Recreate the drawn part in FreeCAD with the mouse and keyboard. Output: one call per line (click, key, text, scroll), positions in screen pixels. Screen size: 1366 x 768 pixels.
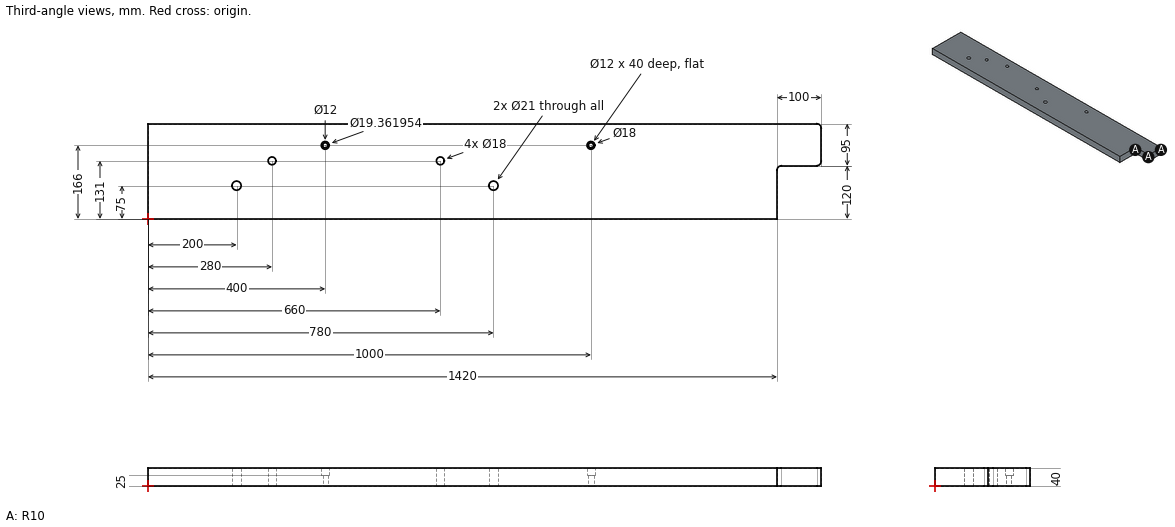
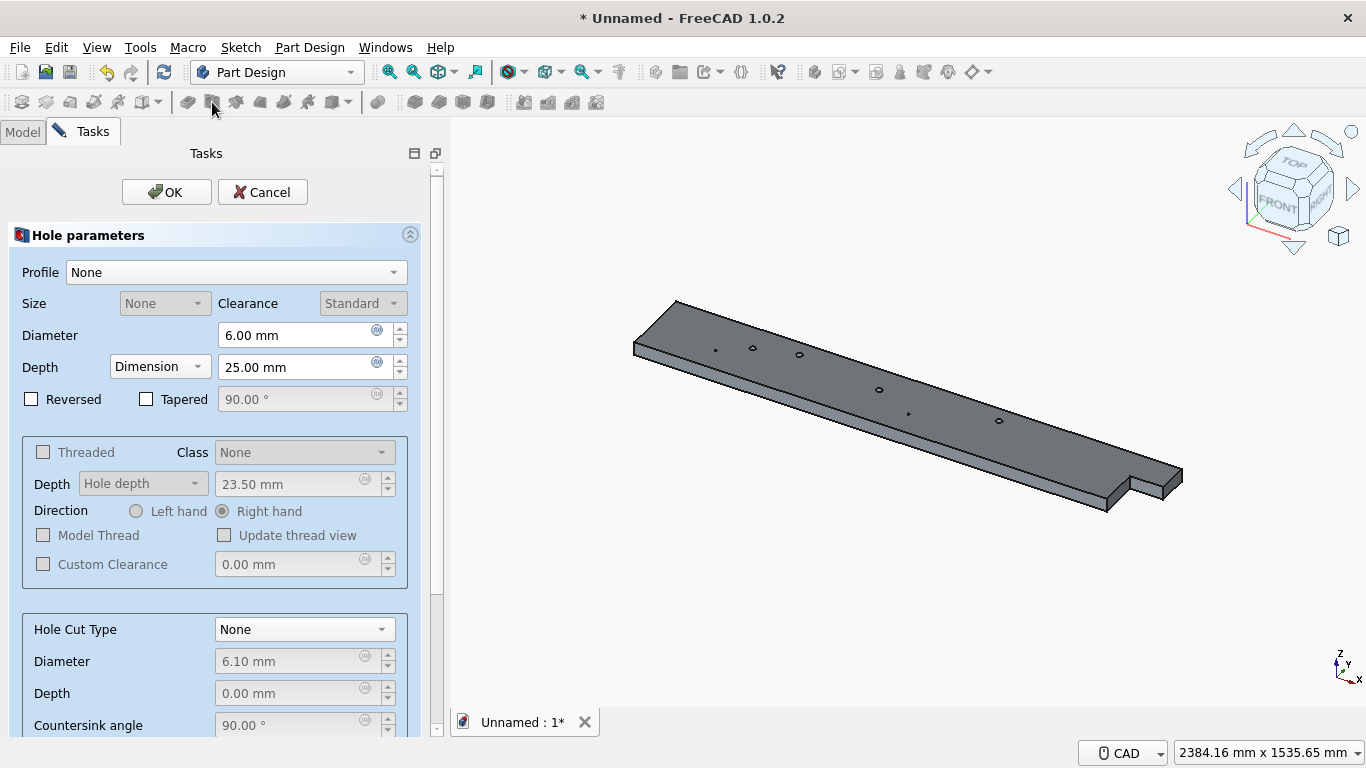
triple_click(305, 335)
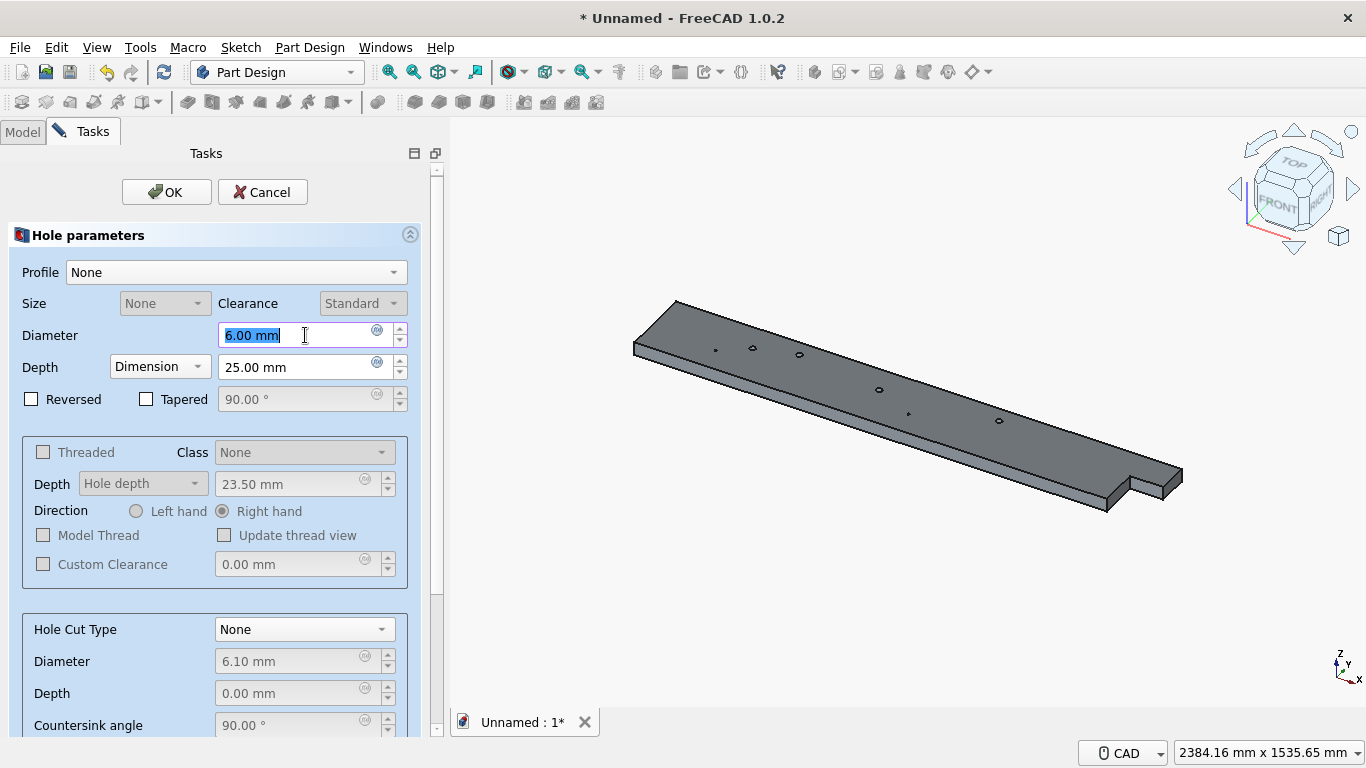
text(21)
key(Tab)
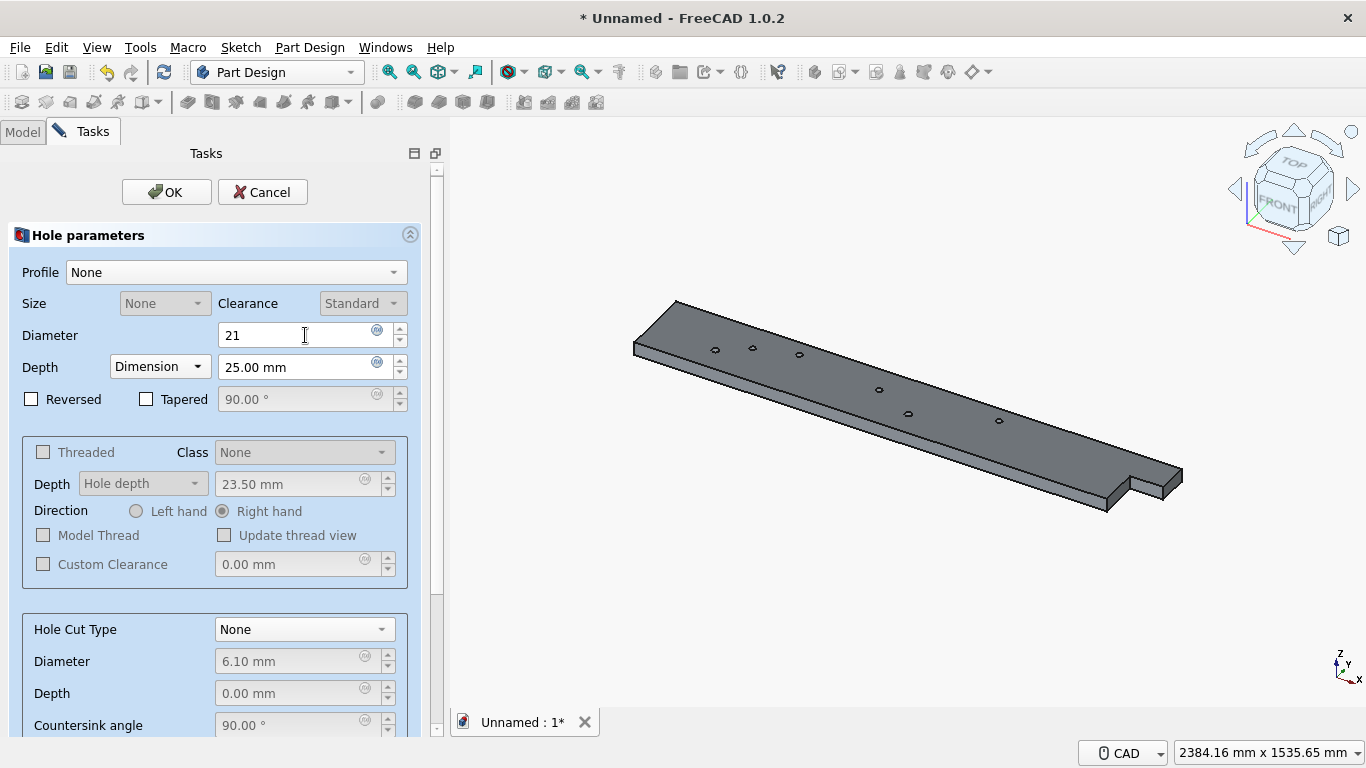
click(161, 366)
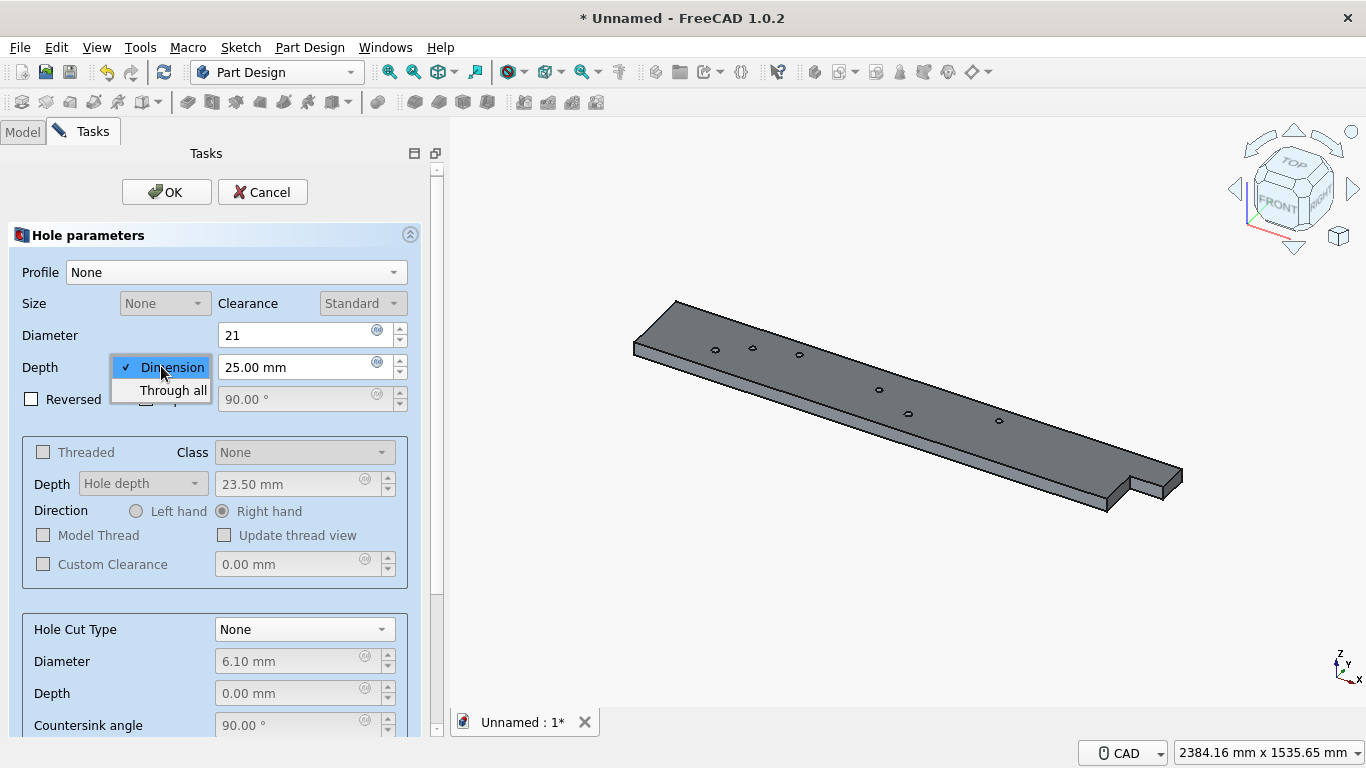
click(160, 390)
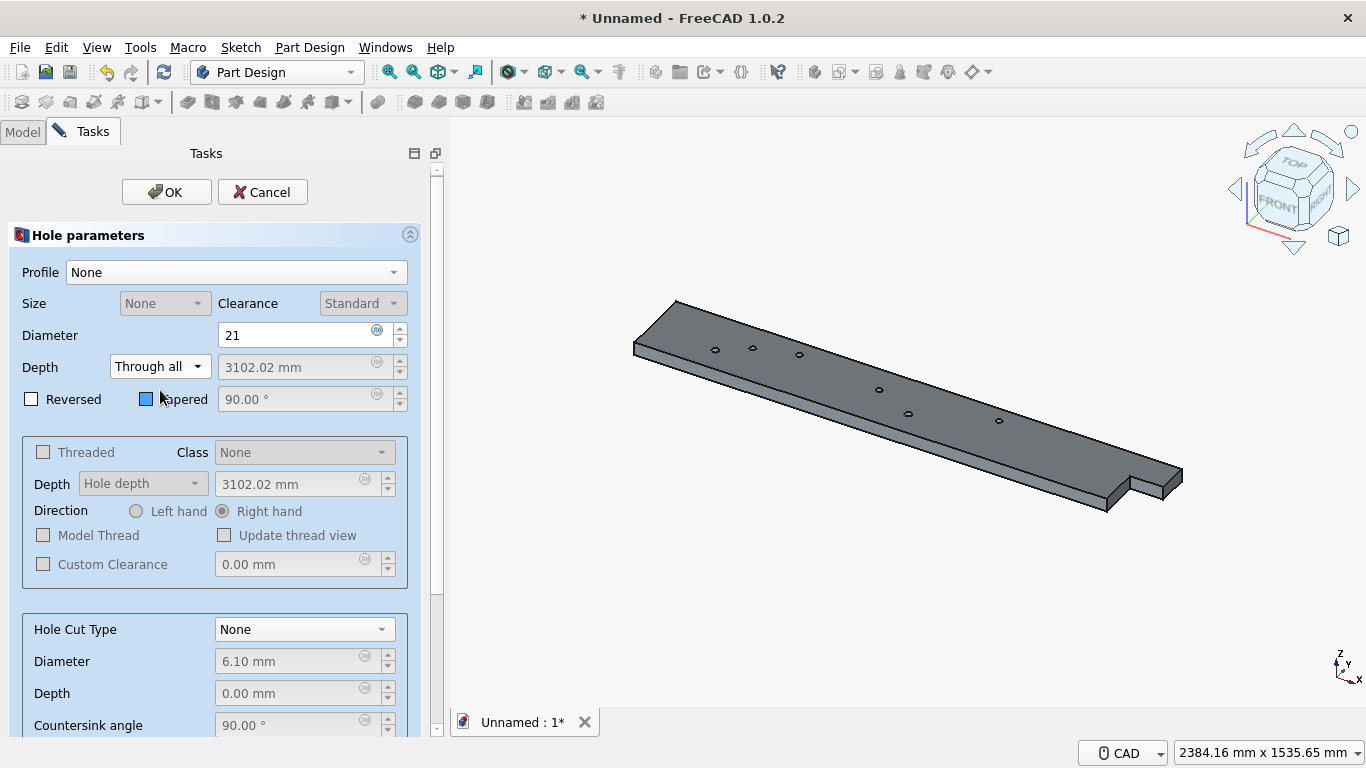
click(167, 192)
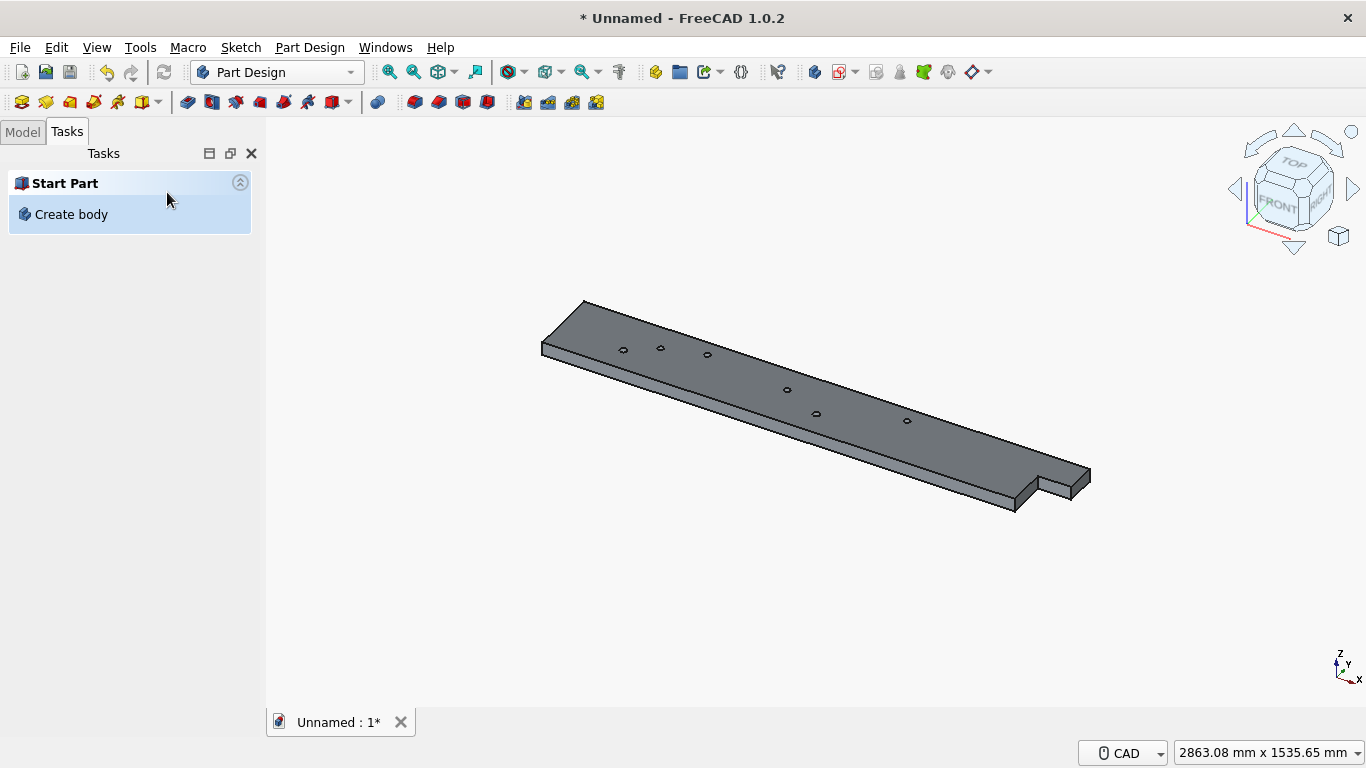
click(1071, 494)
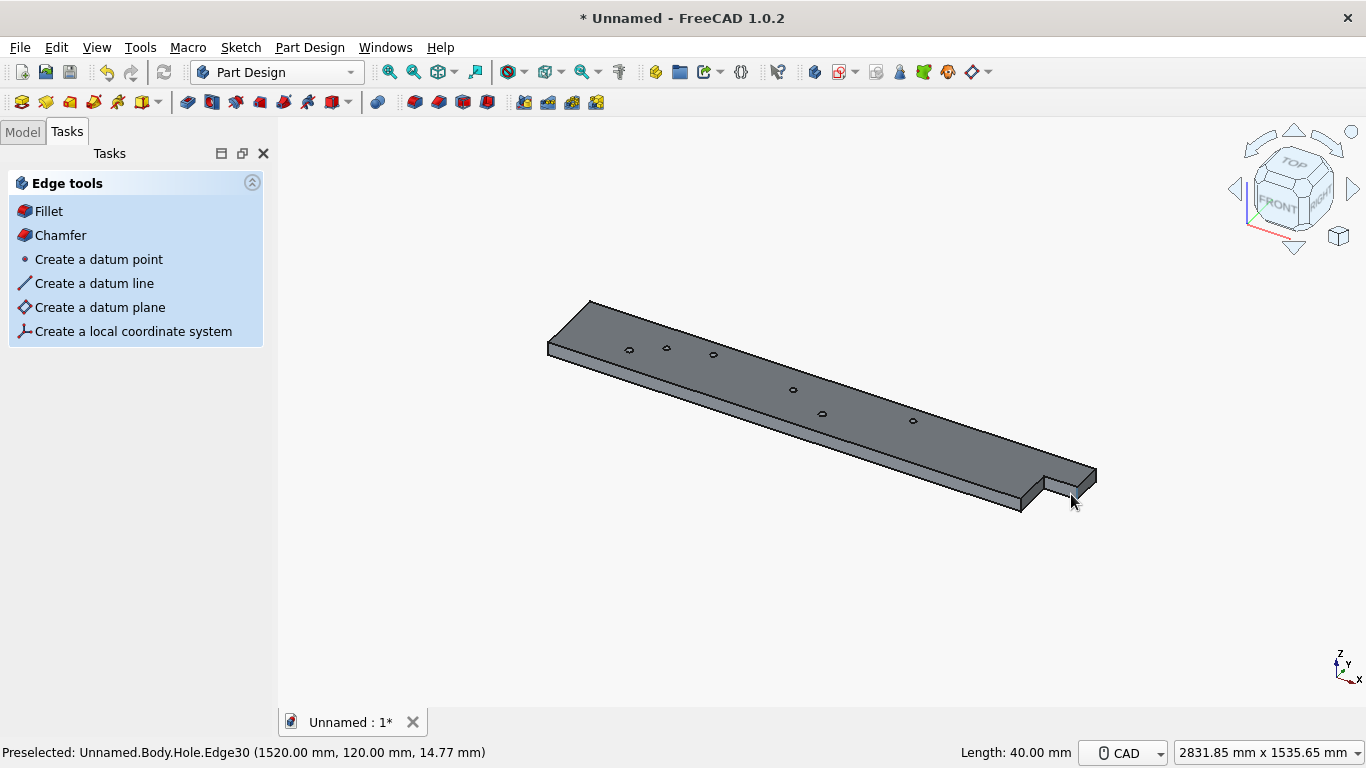
scroll(1096, 474, up, 5)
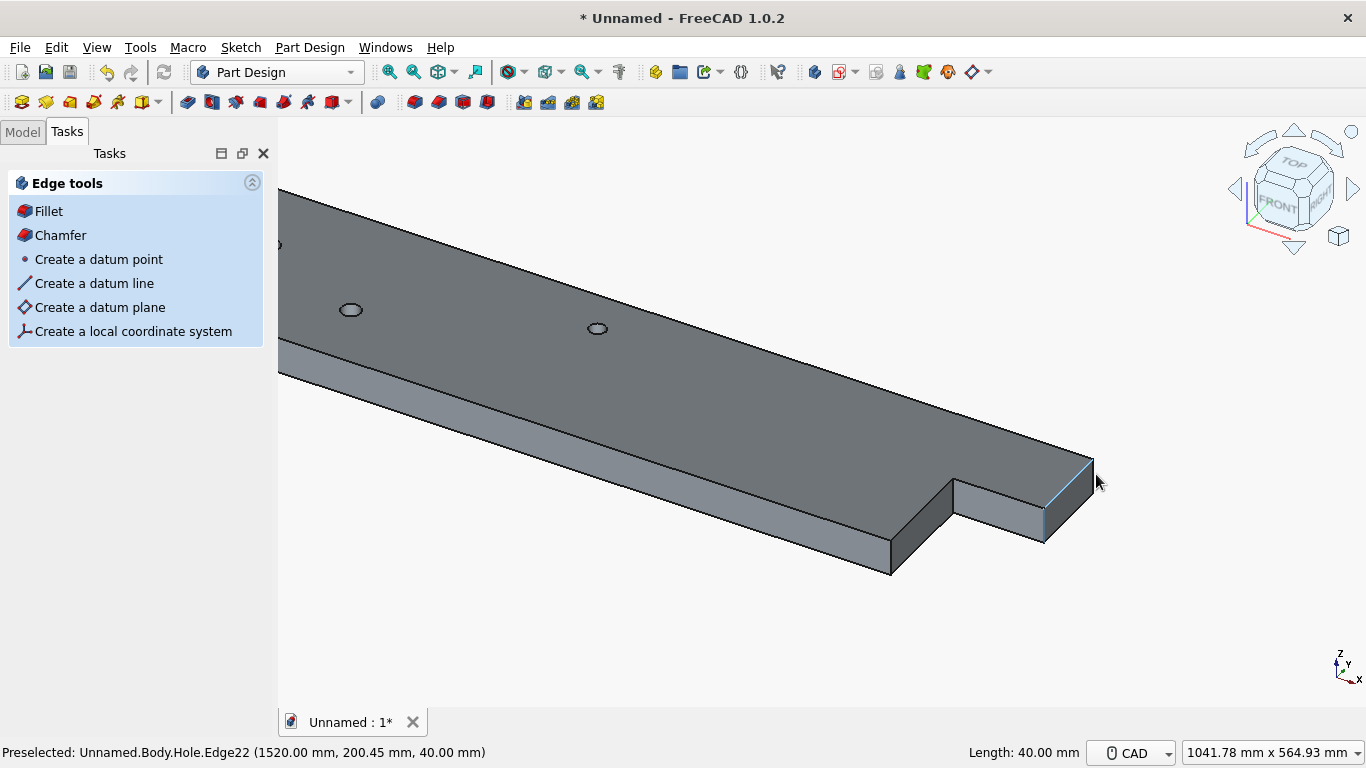
click(390, 72)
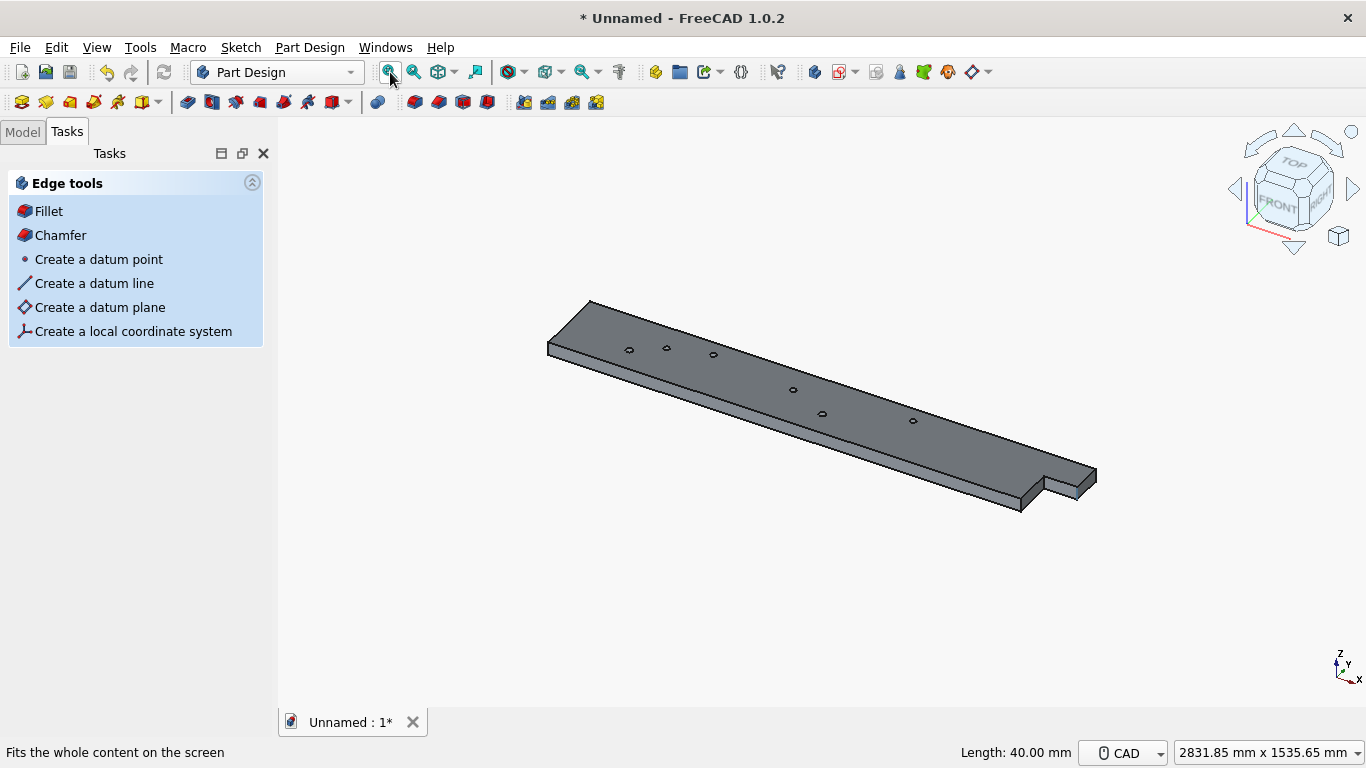
key(0)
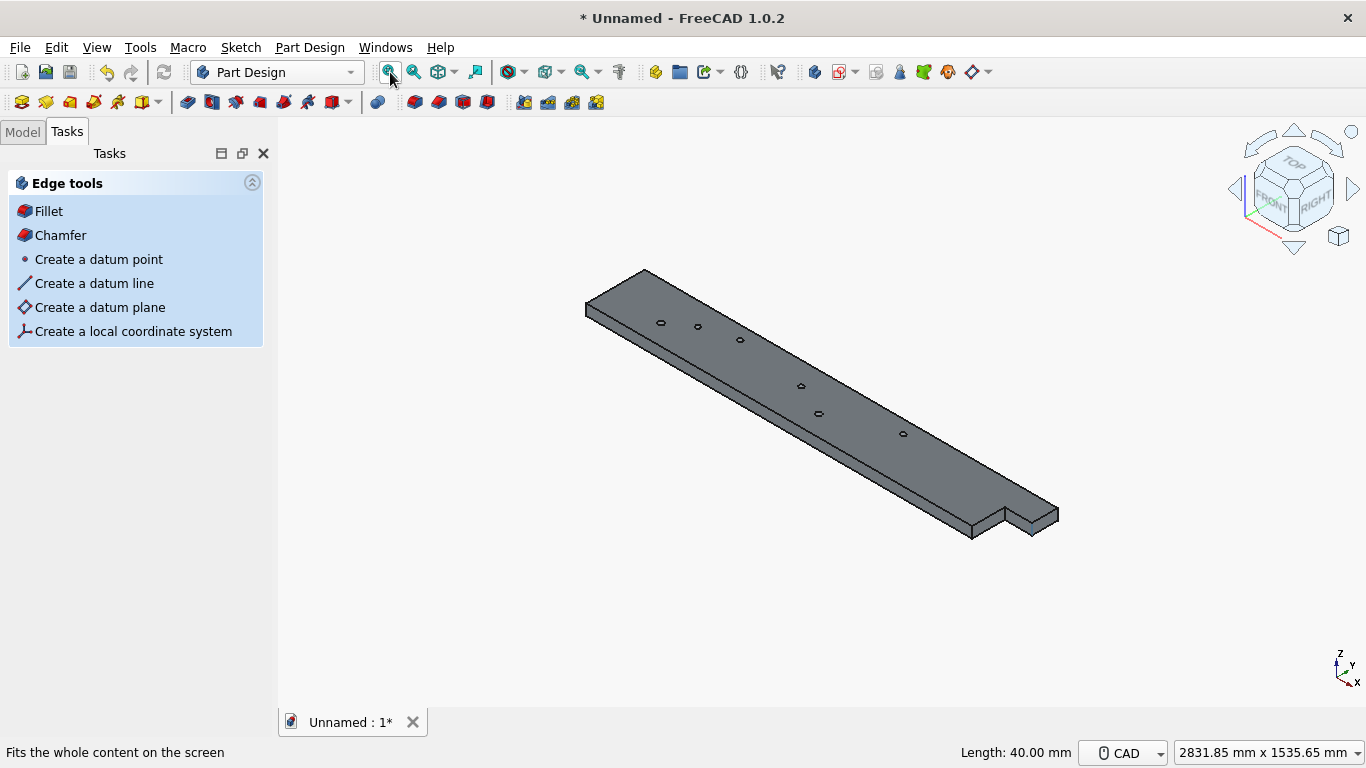
scroll(1058, 513, up, 5)